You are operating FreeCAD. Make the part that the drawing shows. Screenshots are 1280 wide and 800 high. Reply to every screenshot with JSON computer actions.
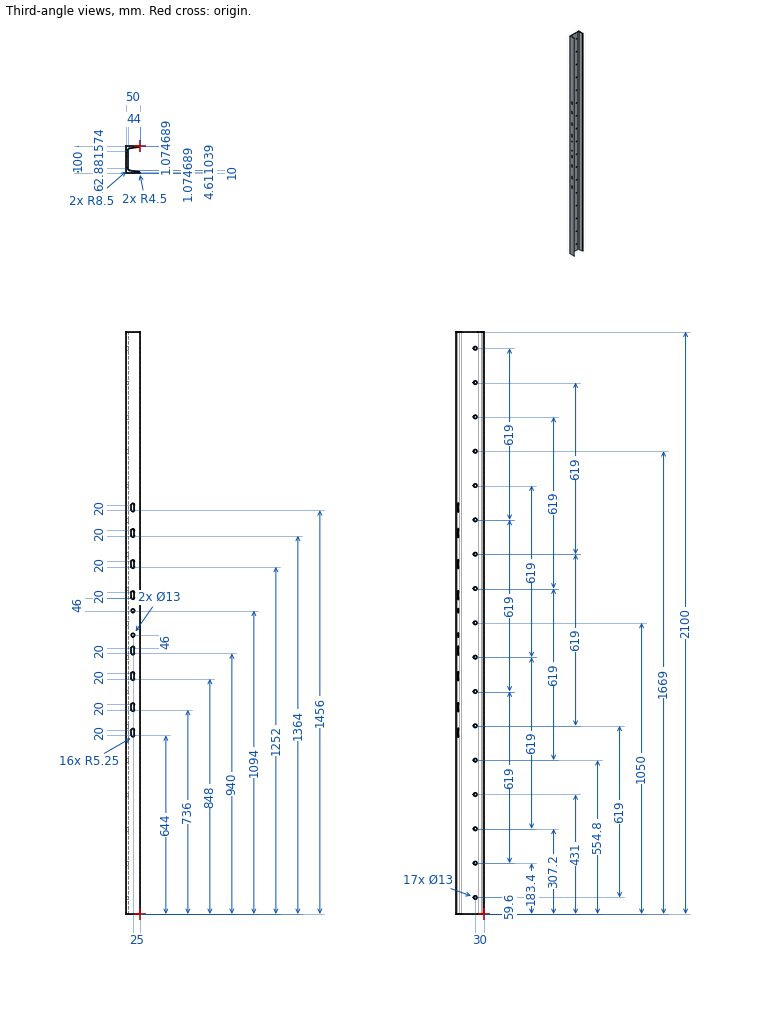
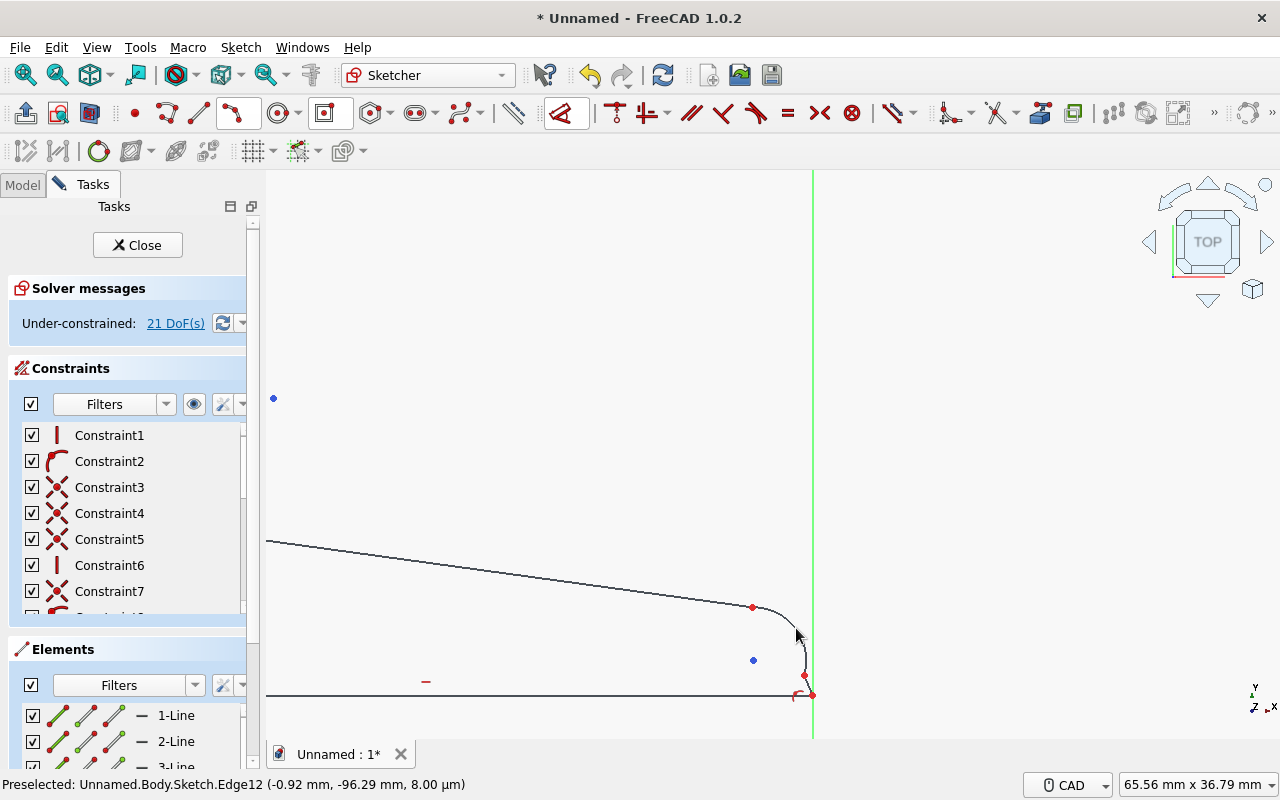
{"action": "scroll", "coordinate": [796, 630], "scroll_direction": "down", "scroll_amount": 7}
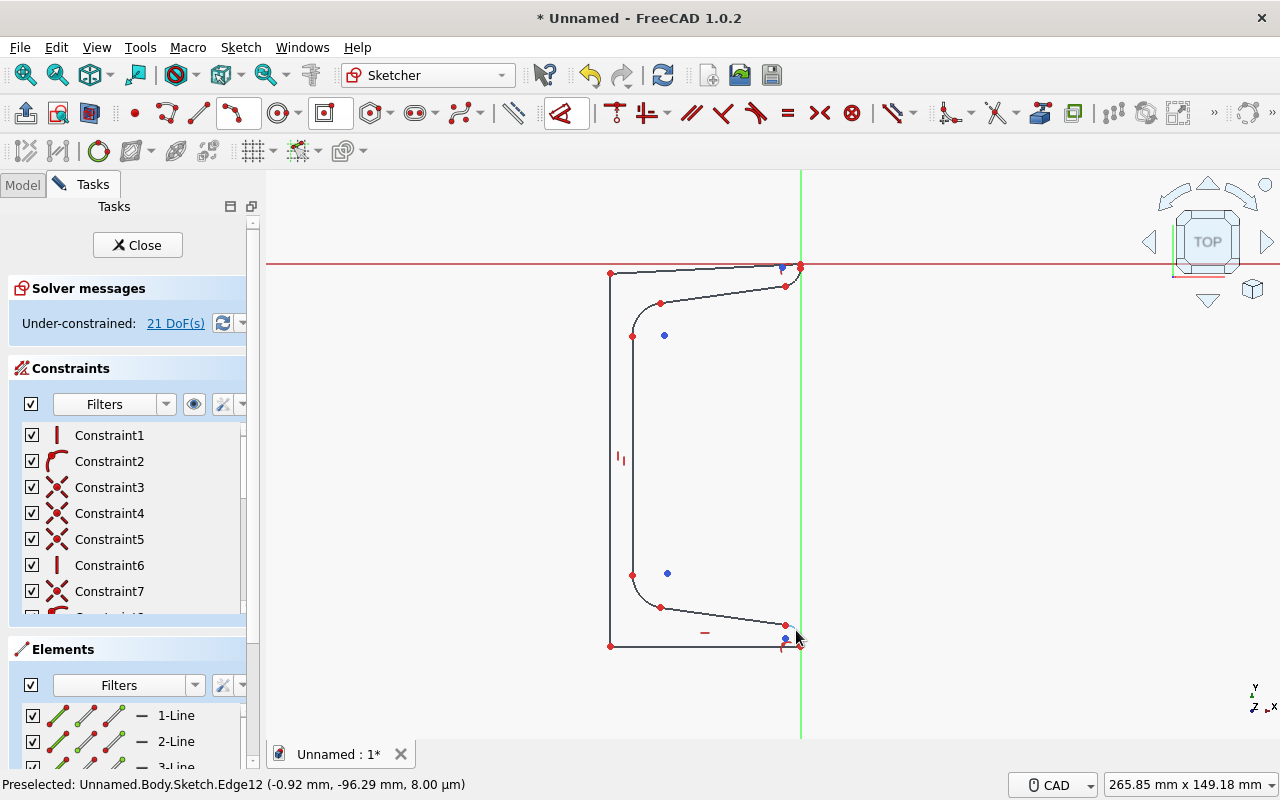
{"action": "left_click", "coordinate": [748, 620]}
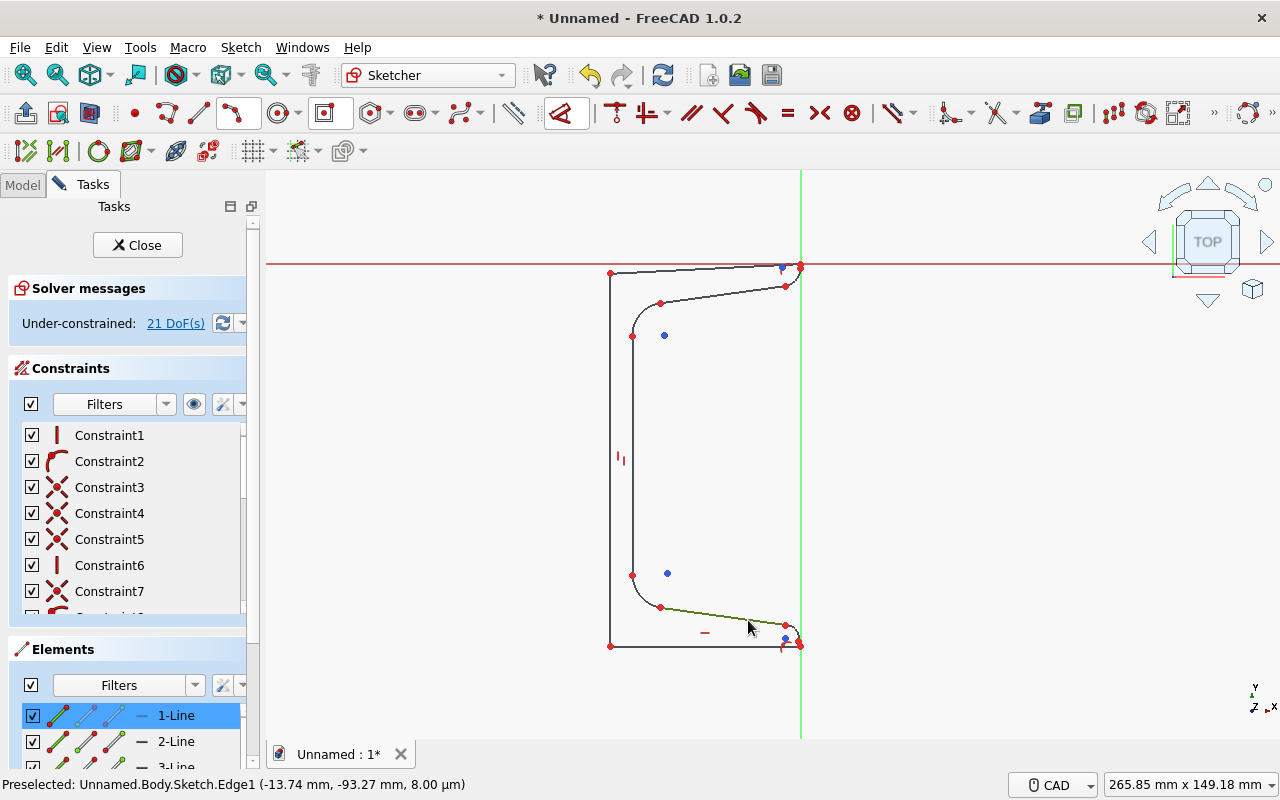
{"action": "left_click", "coordinate": [636, 589]}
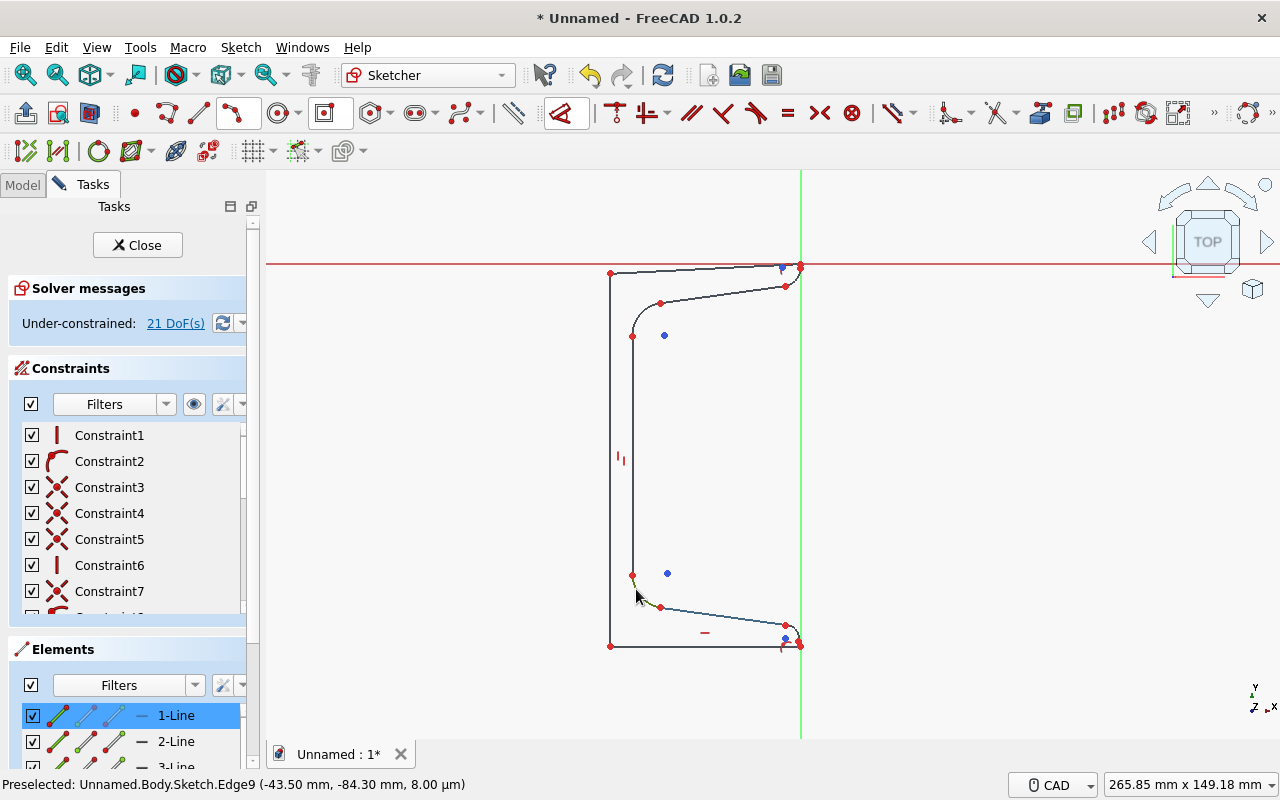
{"action": "left_click", "coordinate": [756, 114]}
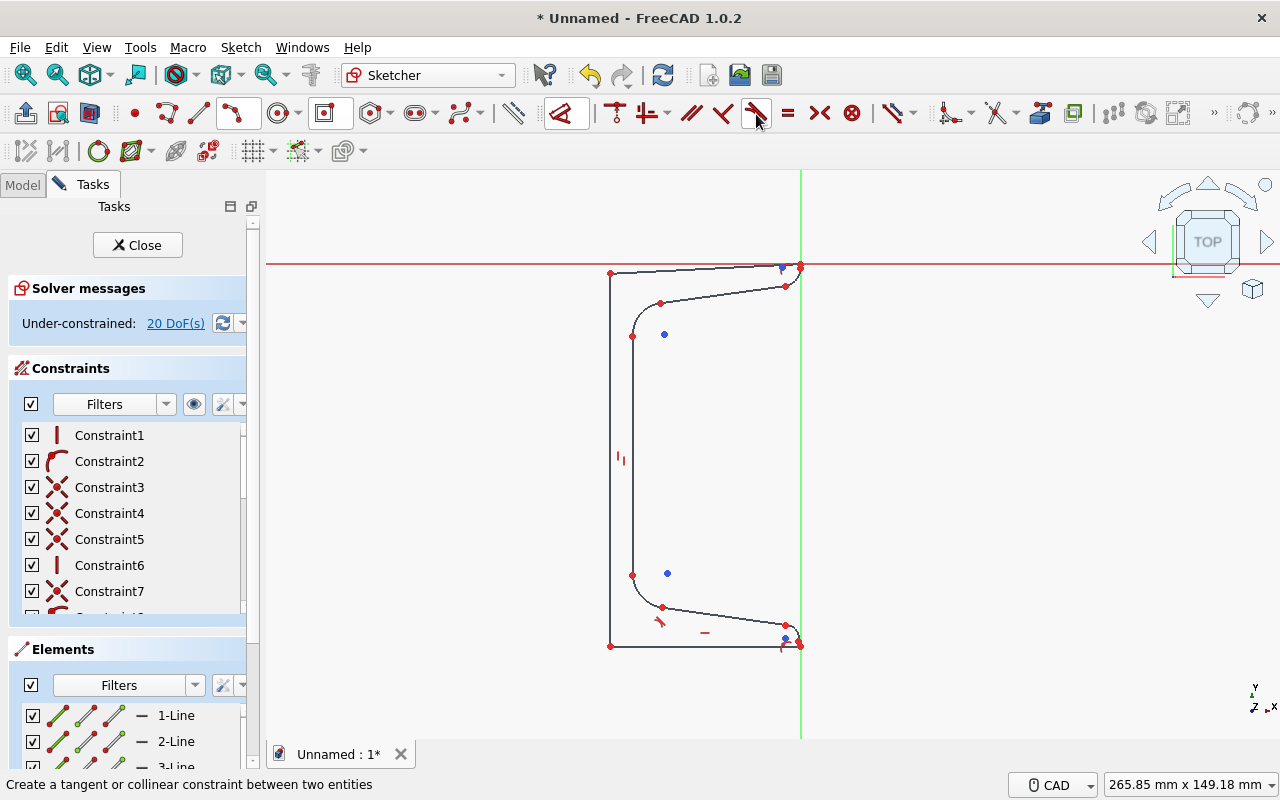
{"action": "left_click", "coordinate": [749, 620]}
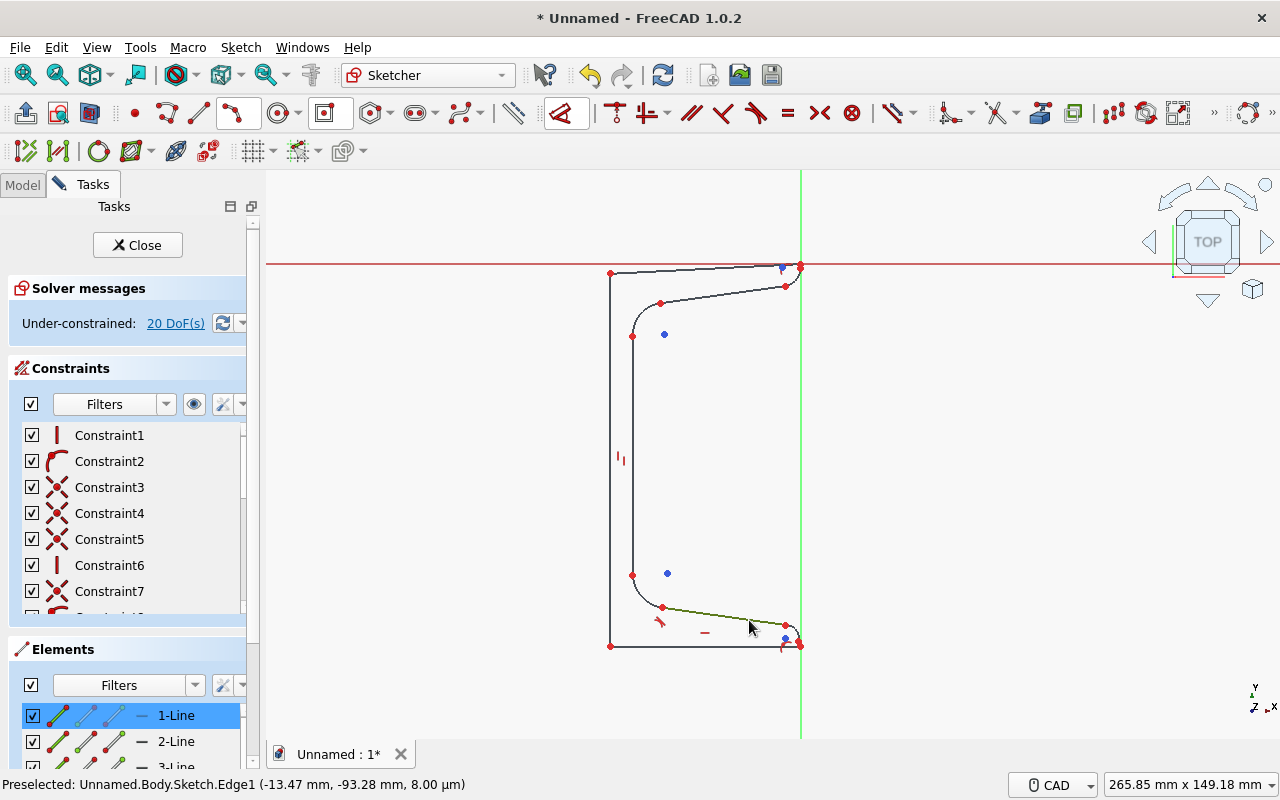
{"action": "scroll", "coordinate": [793, 627], "scroll_direction": "up", "scroll_amount": 4}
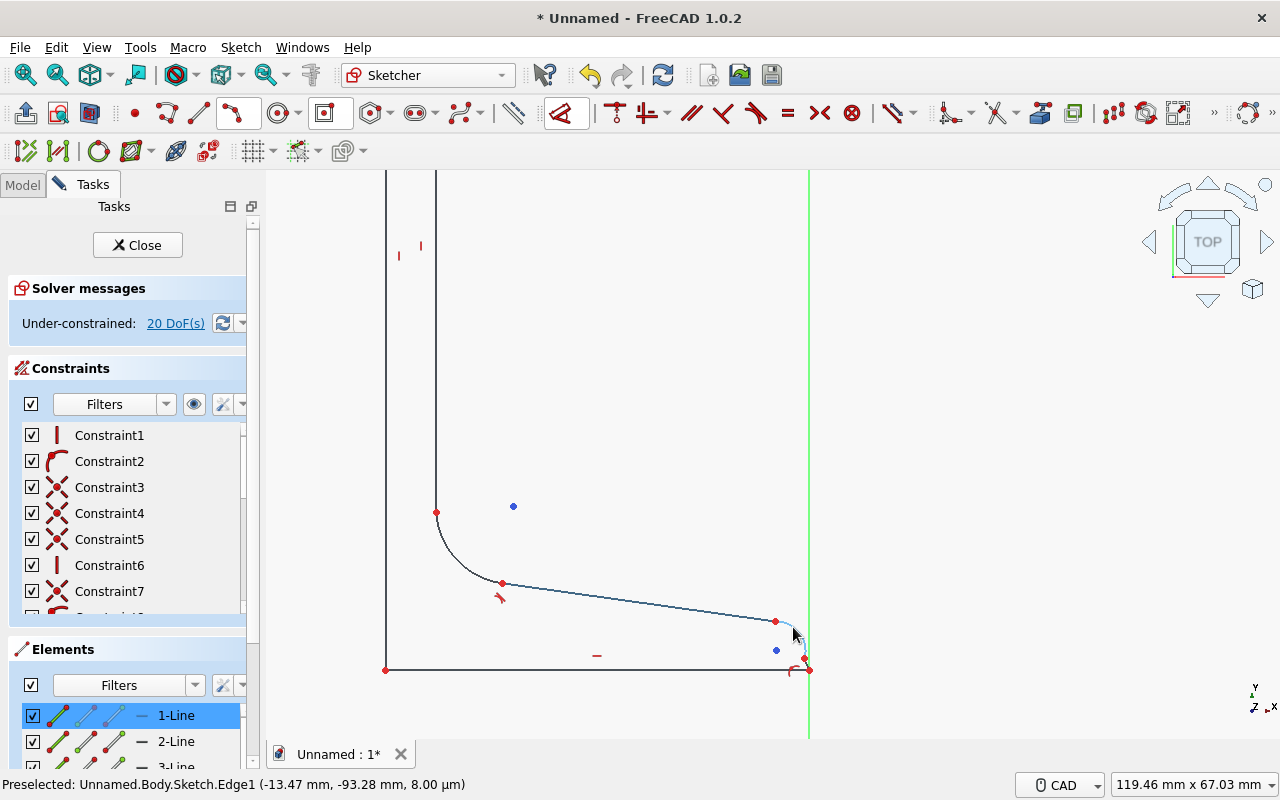
{"action": "left_click", "coordinate": [792, 626]}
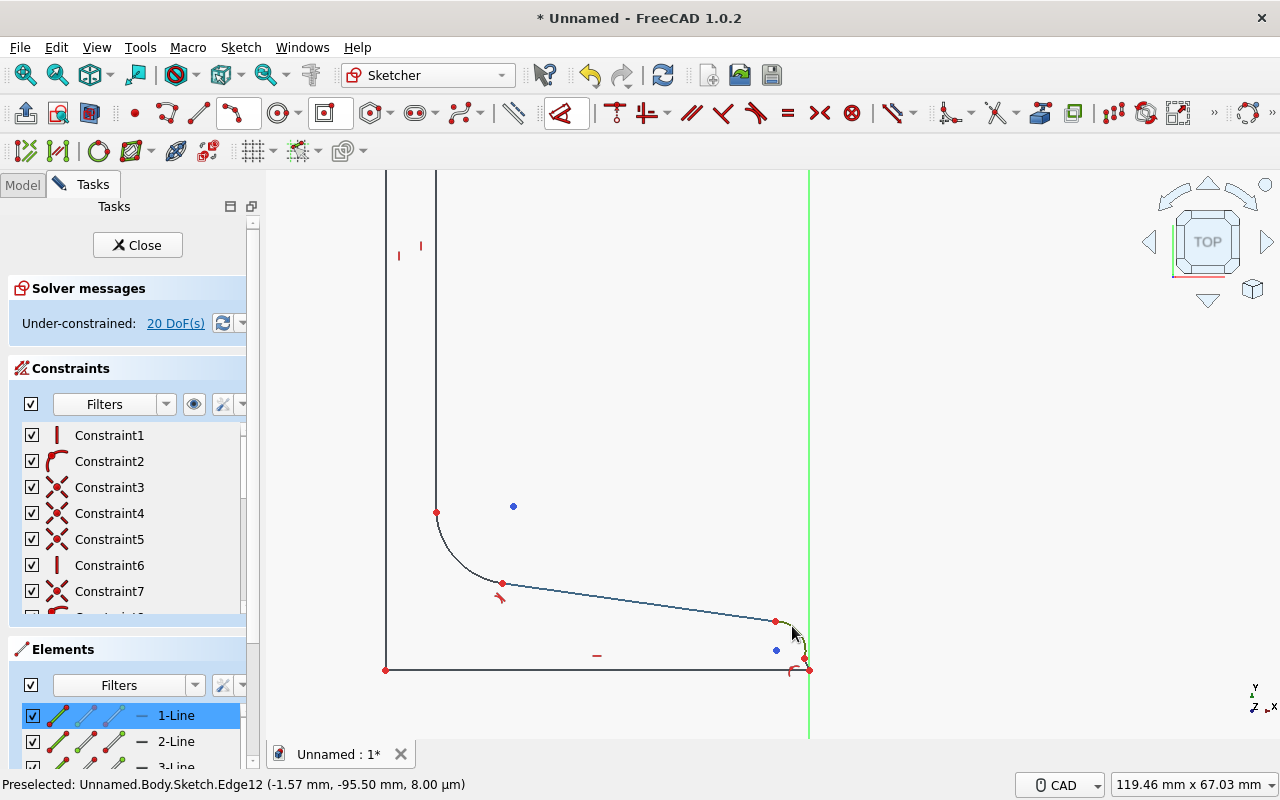
{"action": "left_click", "coordinate": [756, 114]}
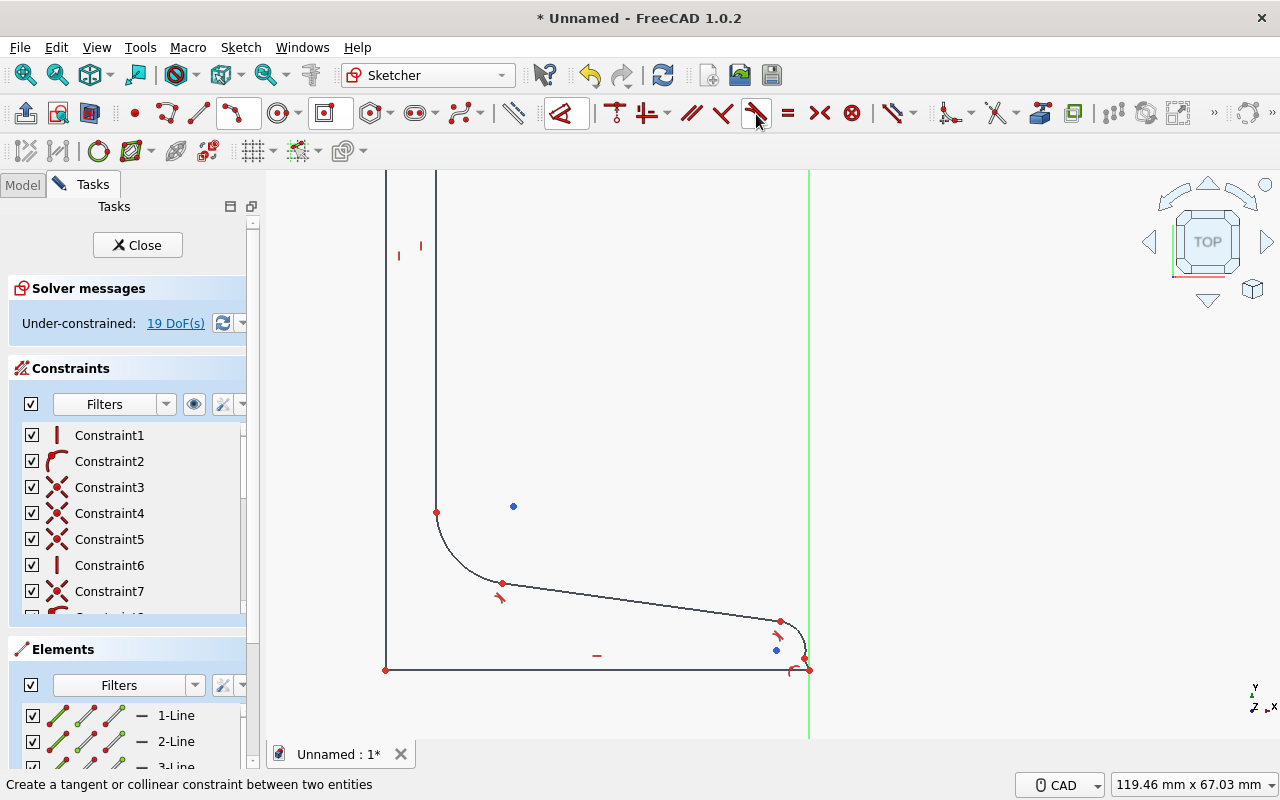
{"action": "left_click", "coordinate": [436, 352]}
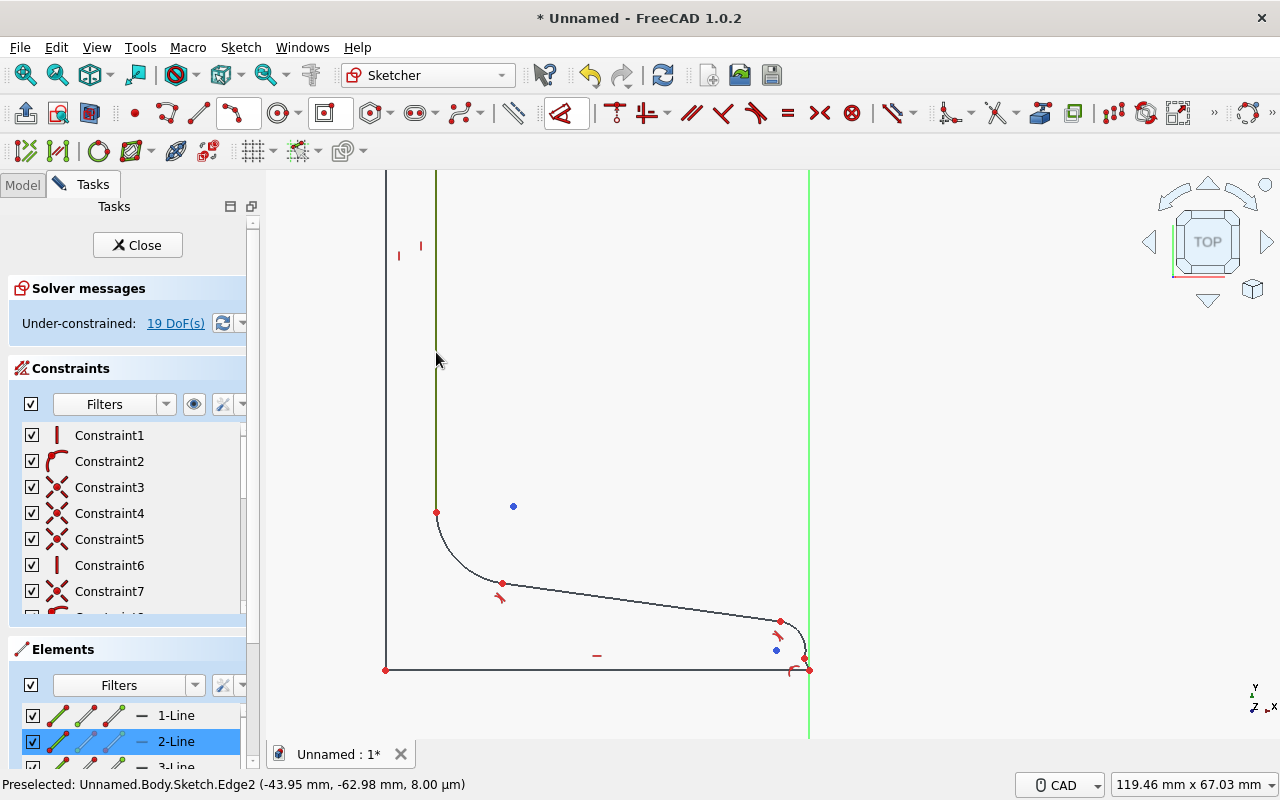
{"action": "left_click", "coordinate": [445, 542]}